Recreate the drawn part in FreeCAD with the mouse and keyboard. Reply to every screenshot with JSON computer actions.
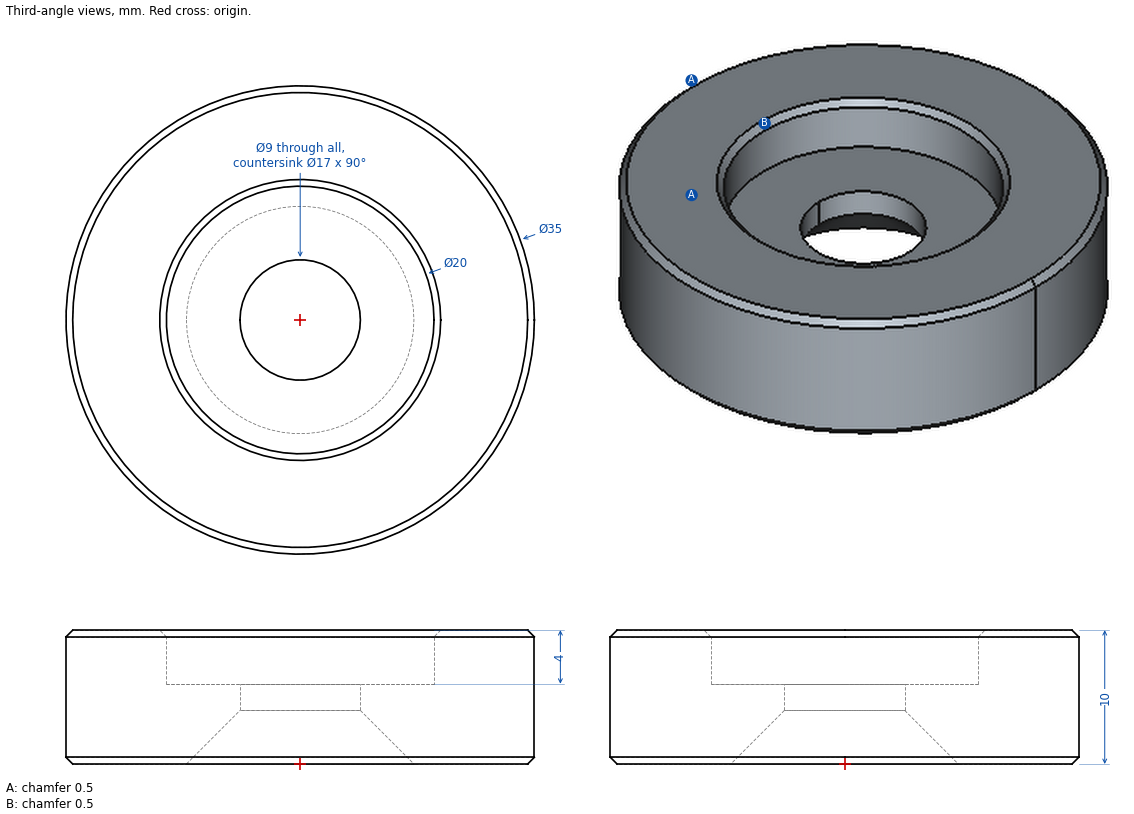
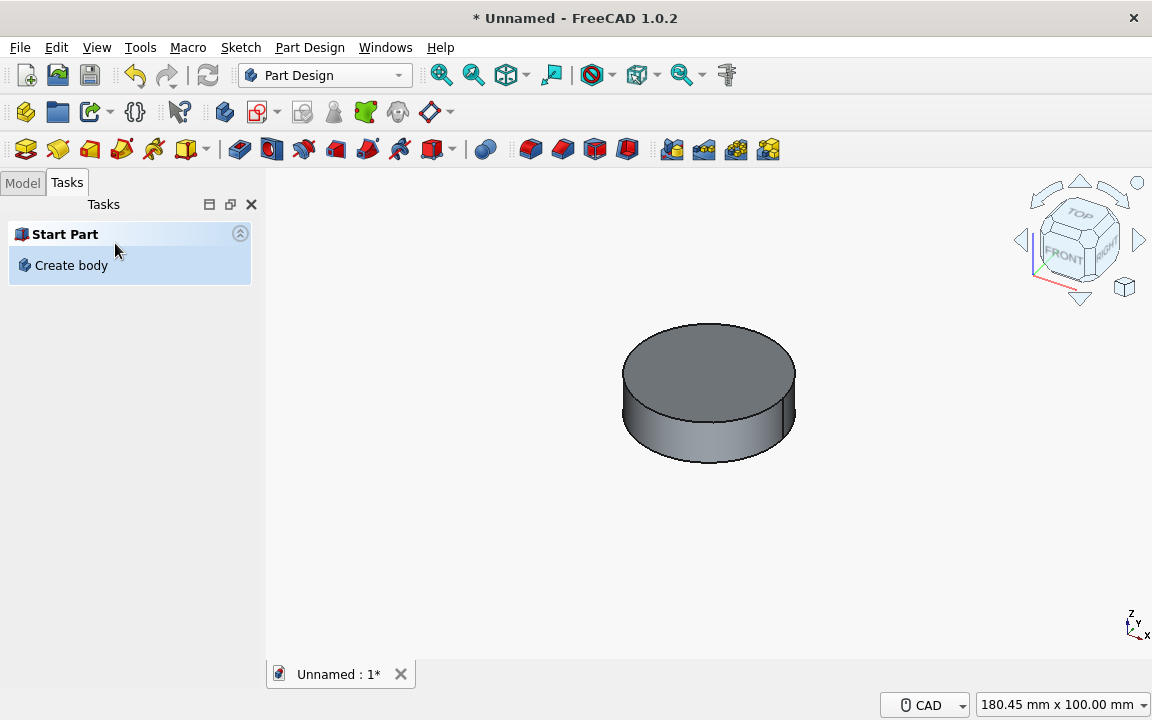
{"action": "left_click", "coordinate": [442, 76]}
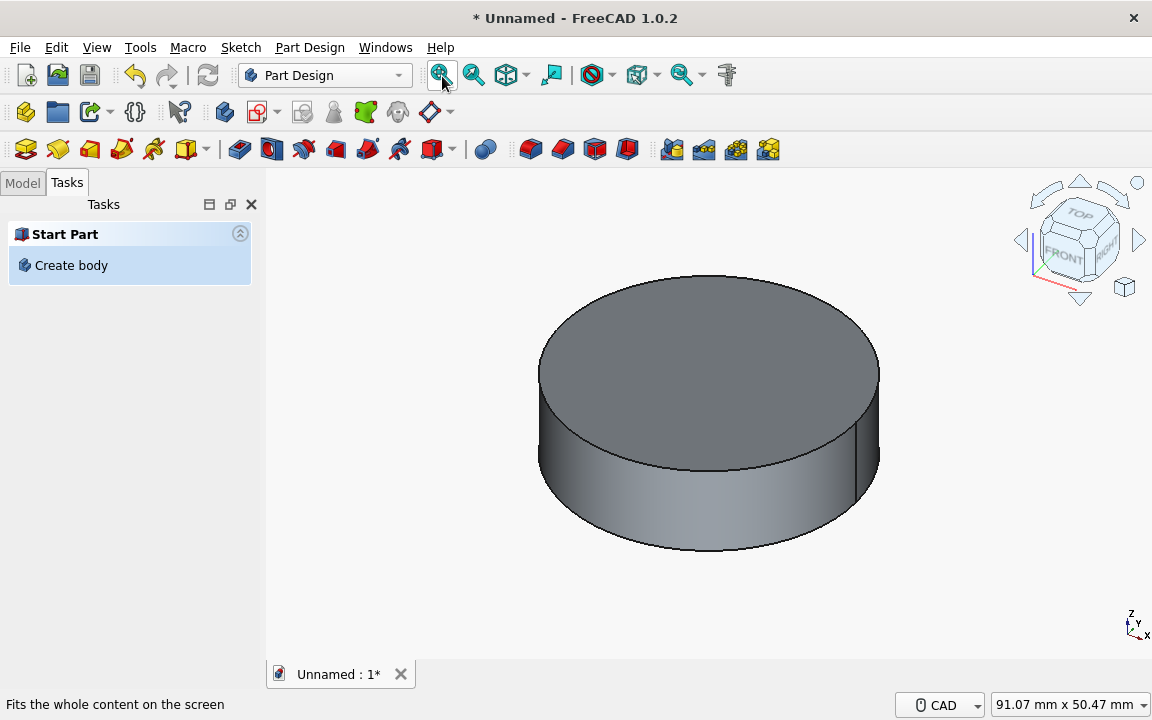
{"action": "left_click", "coordinate": [540, 383]}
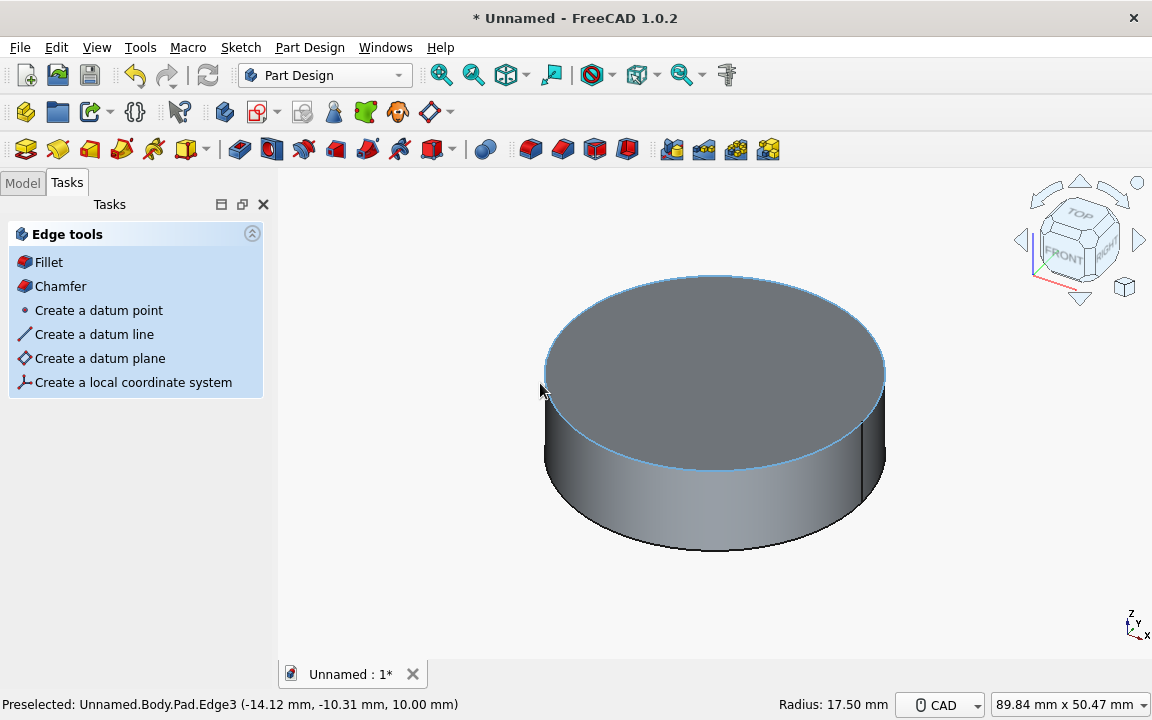
{"action": "key", "text": "0"}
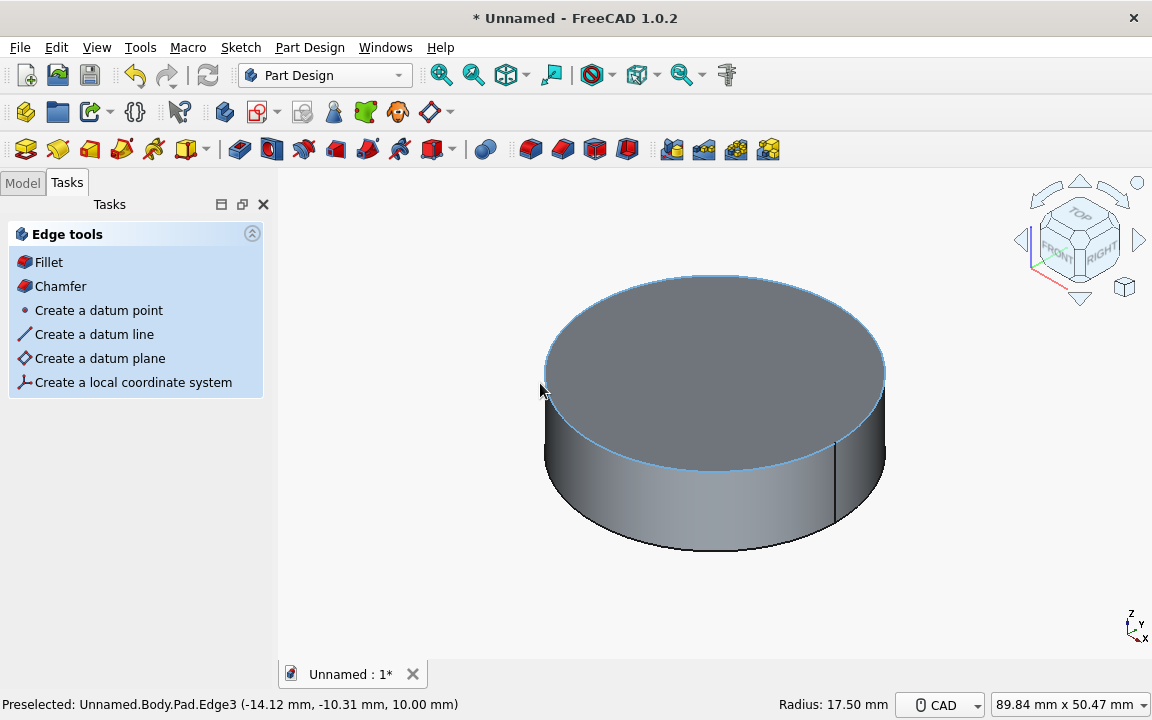
{"action": "key", "text": "2"}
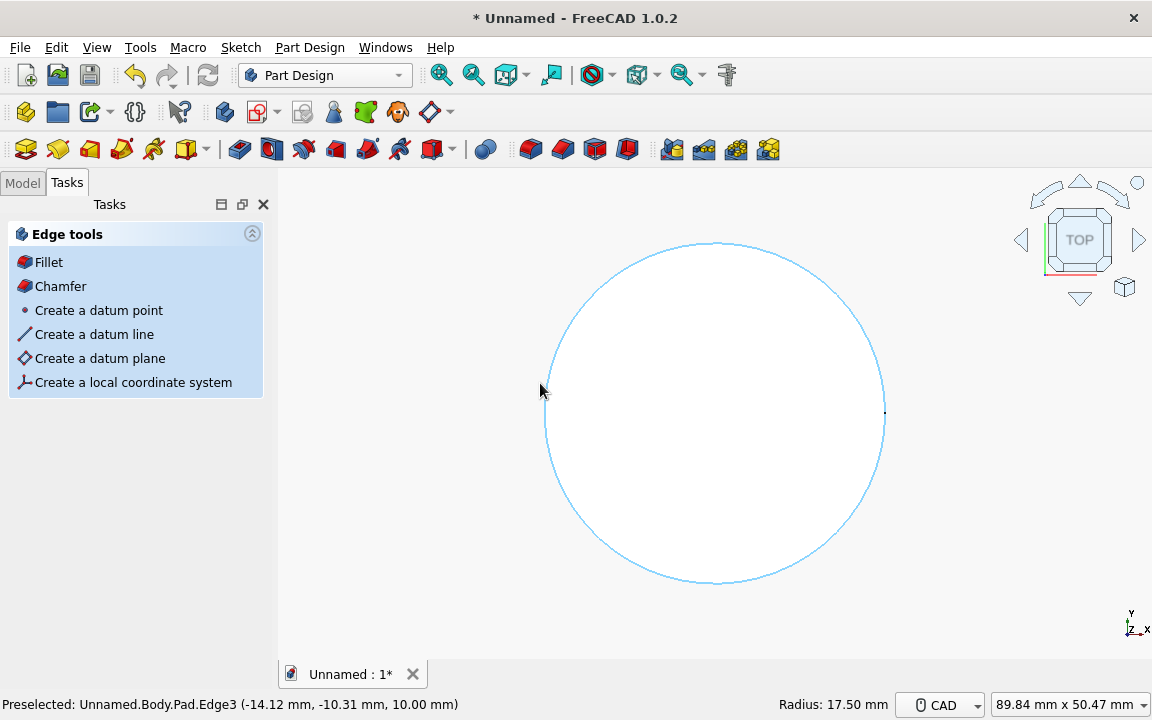
{"action": "key", "text": "1"}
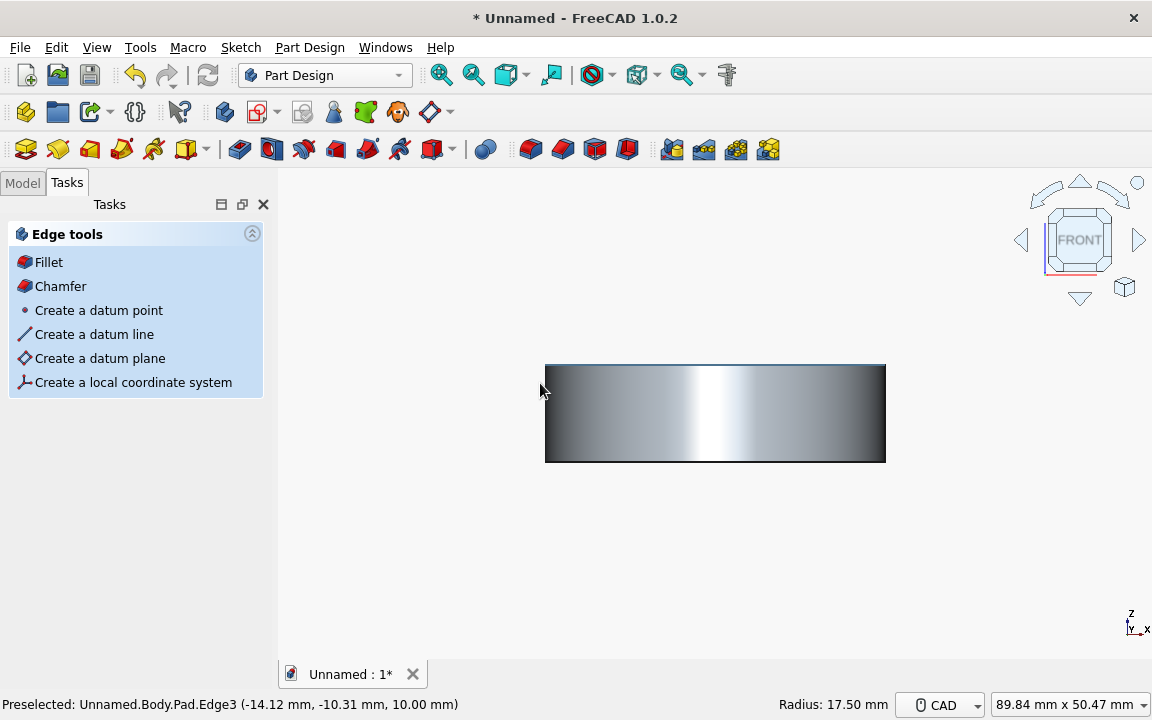
{"action": "left_click", "coordinate": [442, 76]}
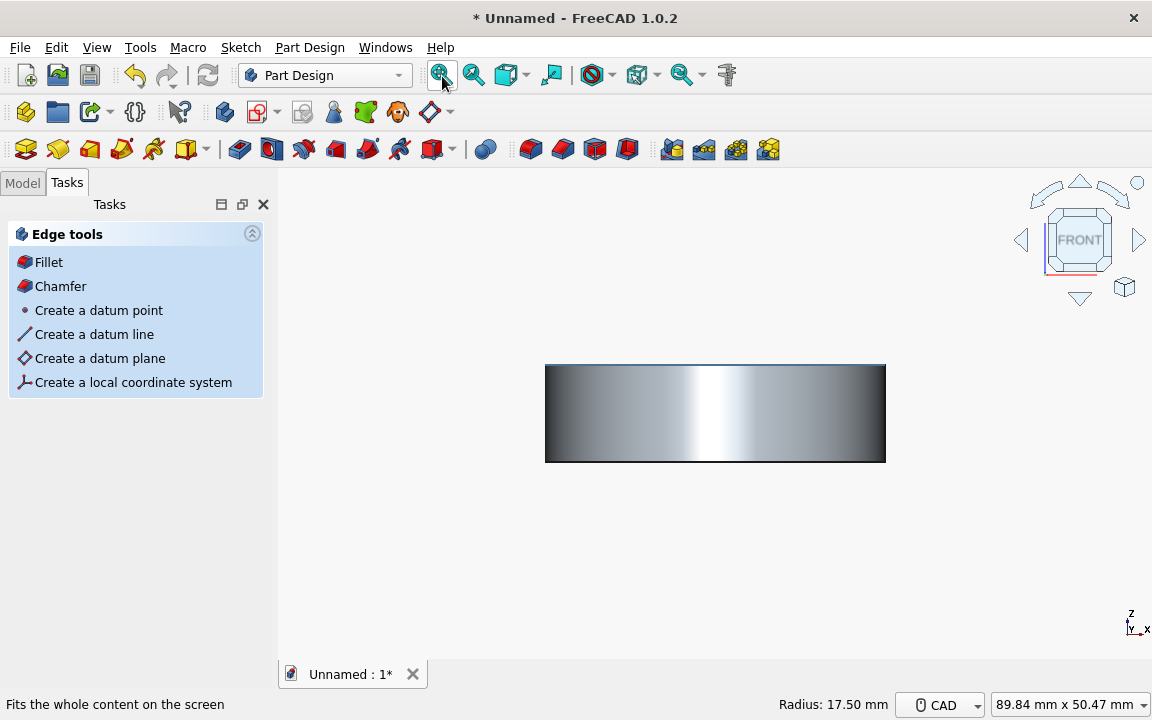
{"action": "left_click", "coordinate": [577, 461], "text": "ctrl"}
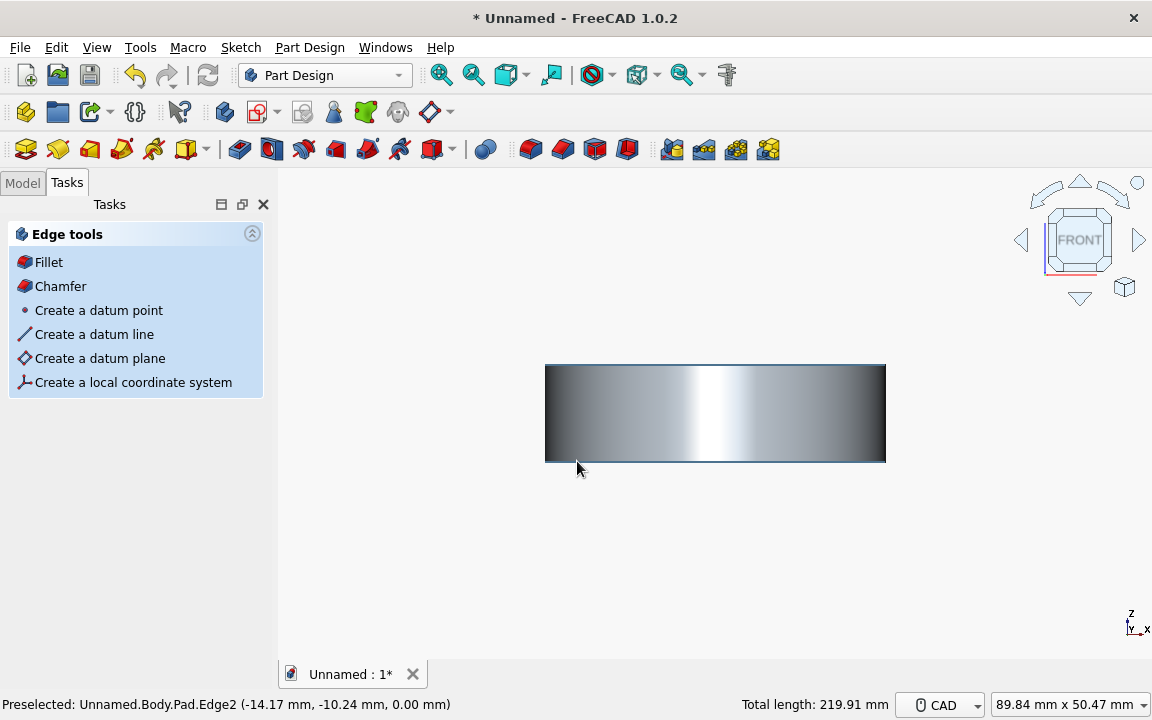
{"action": "left_click", "coordinate": [564, 150]}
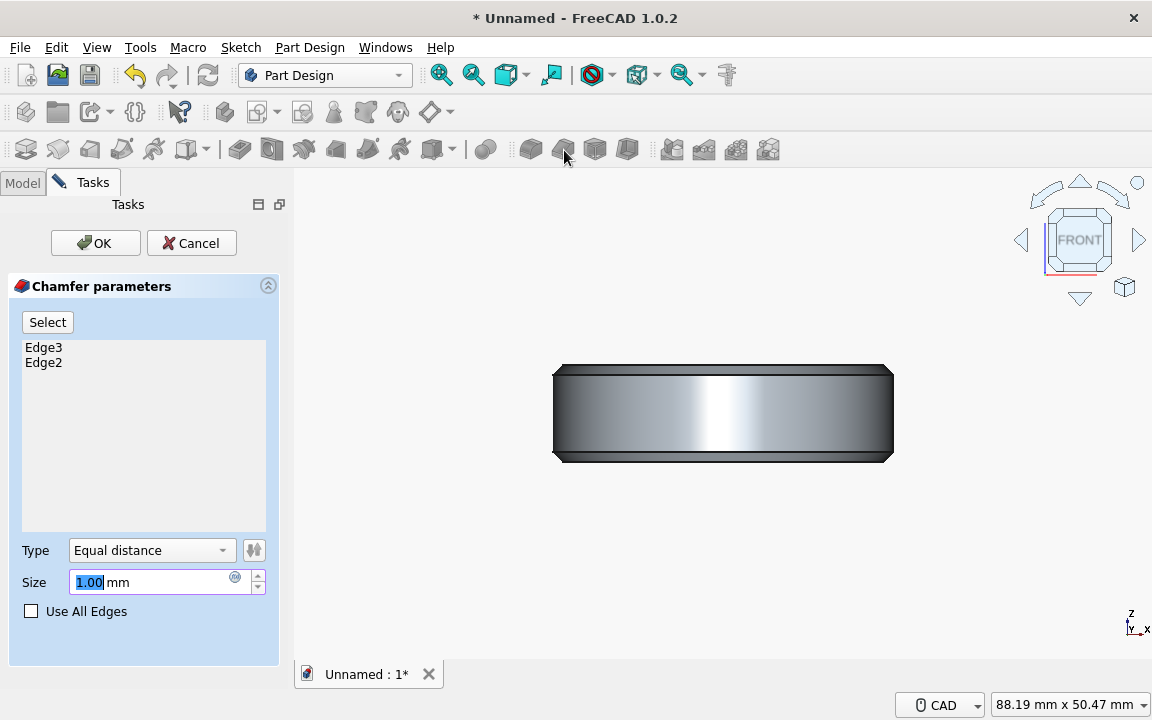
{"action": "type", "text": "0.5"}
{"action": "key", "text": "Tab"}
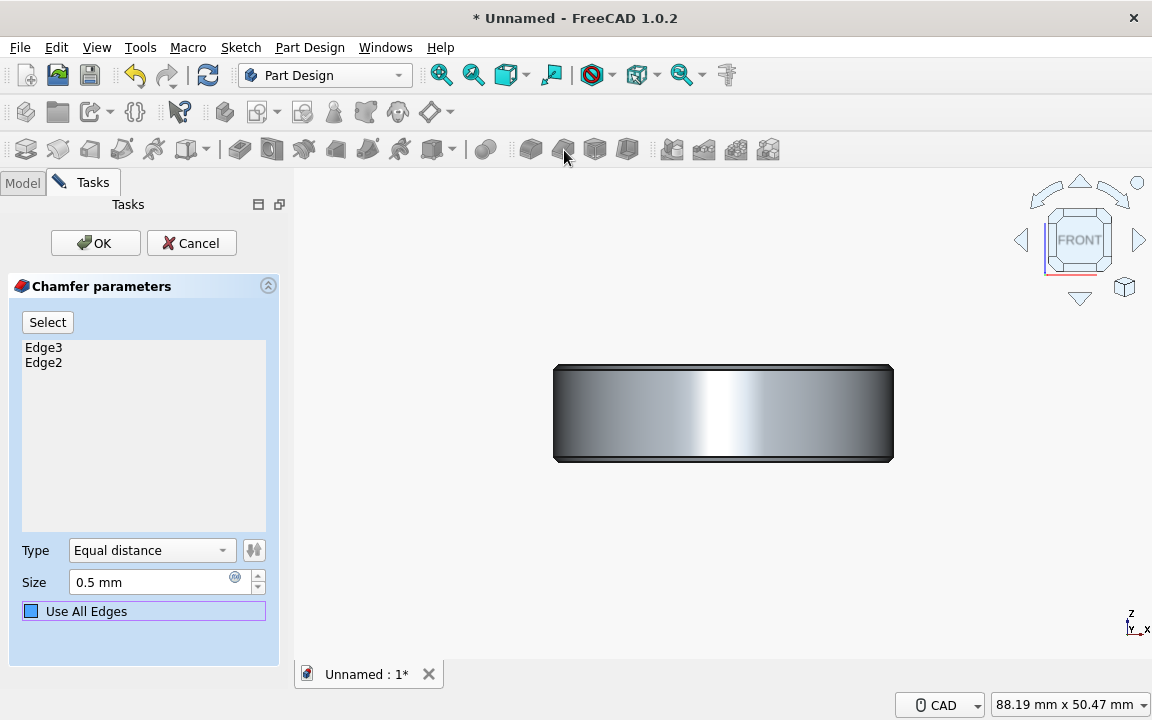
{"action": "left_click", "coordinate": [96, 243]}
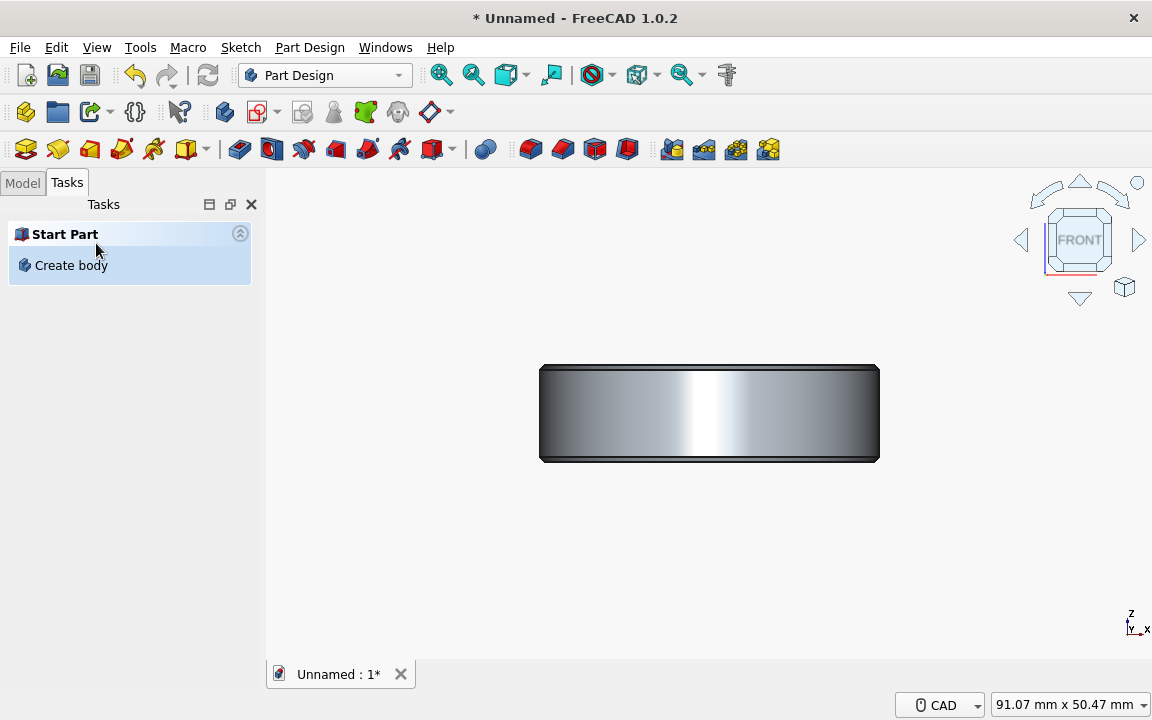
{"action": "left_click", "coordinate": [442, 76]}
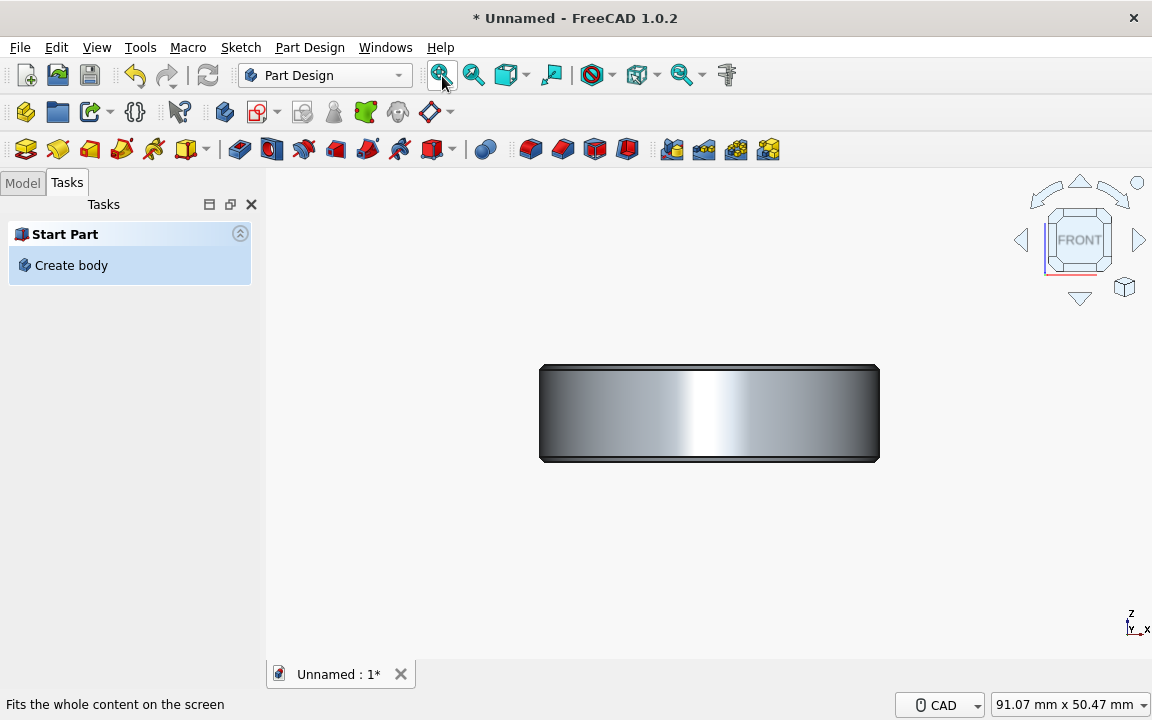
{"action": "left_click", "coordinate": [258, 112]}